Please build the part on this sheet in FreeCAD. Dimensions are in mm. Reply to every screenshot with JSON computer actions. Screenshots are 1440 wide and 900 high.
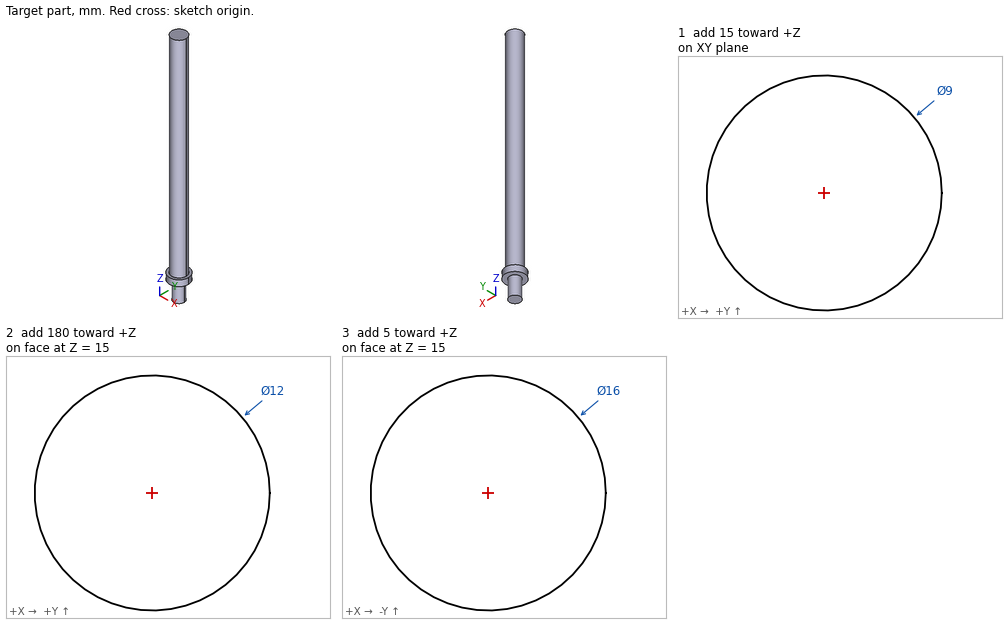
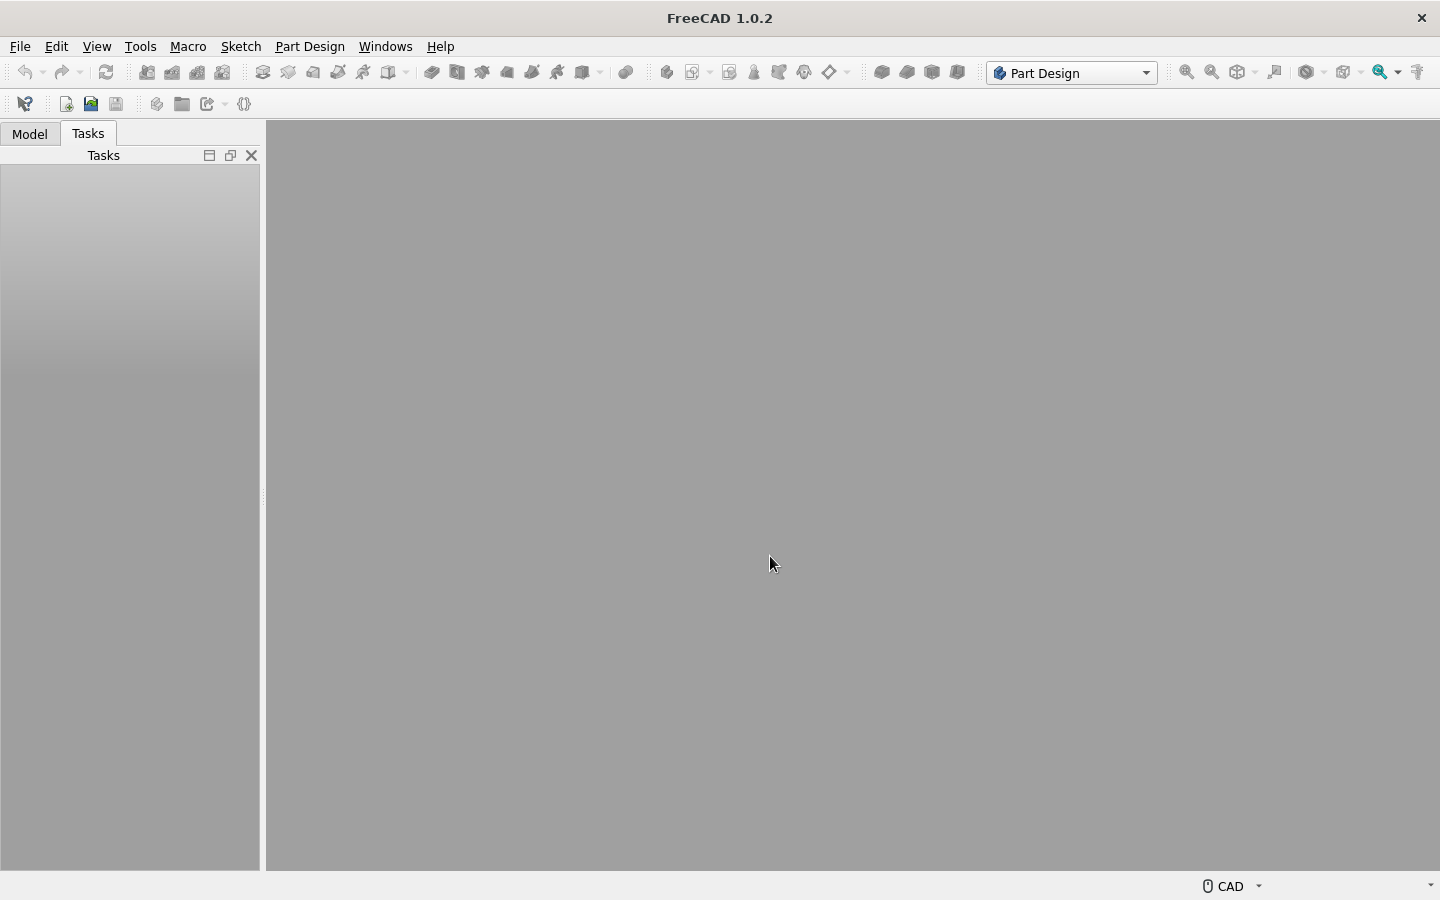
{"action": "key", "text": "ctrl+n"}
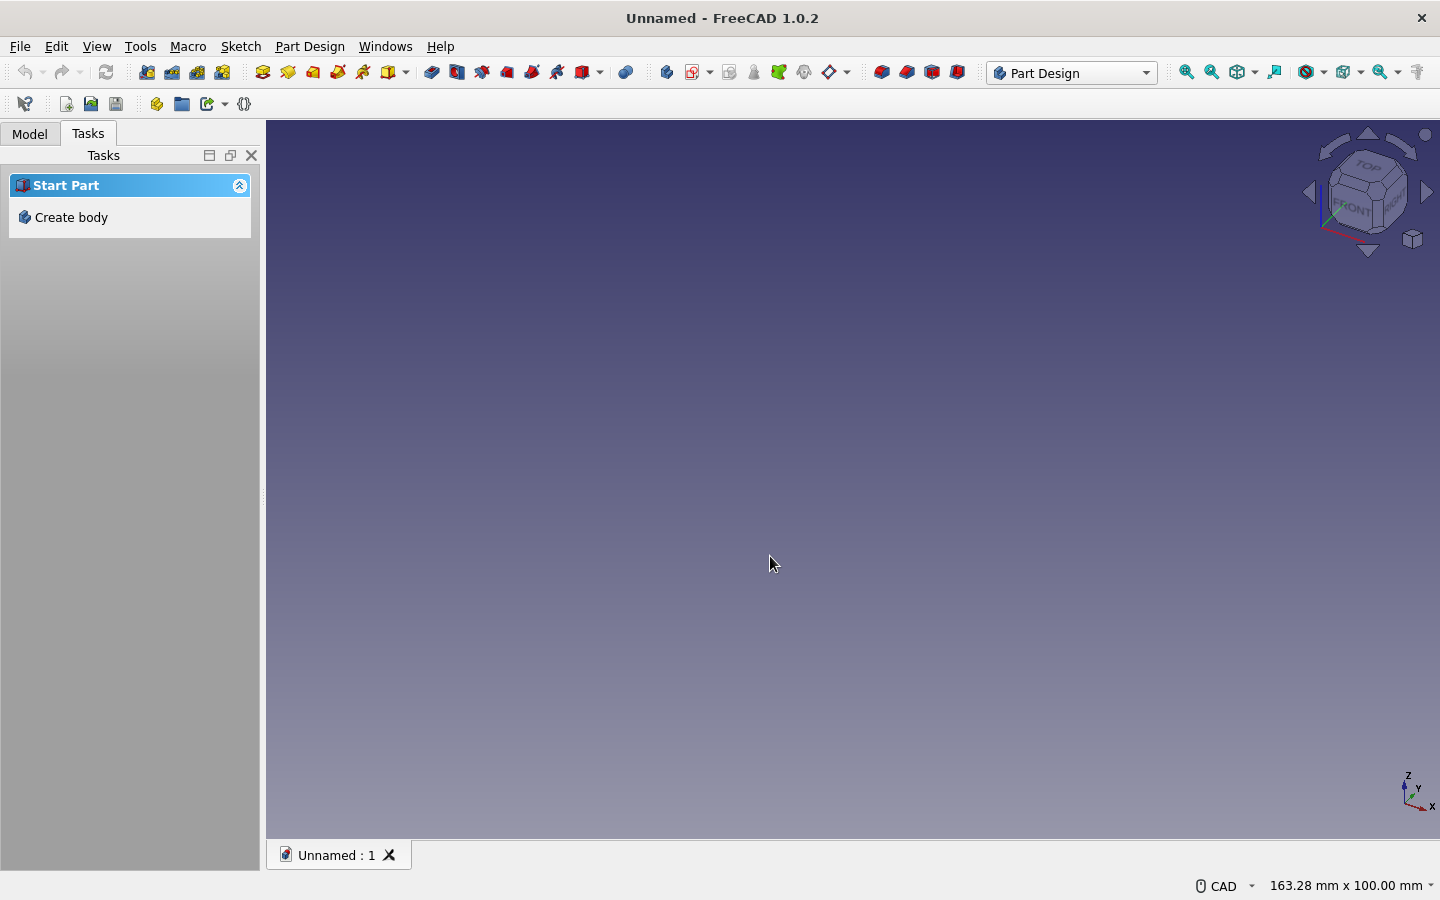
{"action": "left_click", "coordinate": [692, 72]}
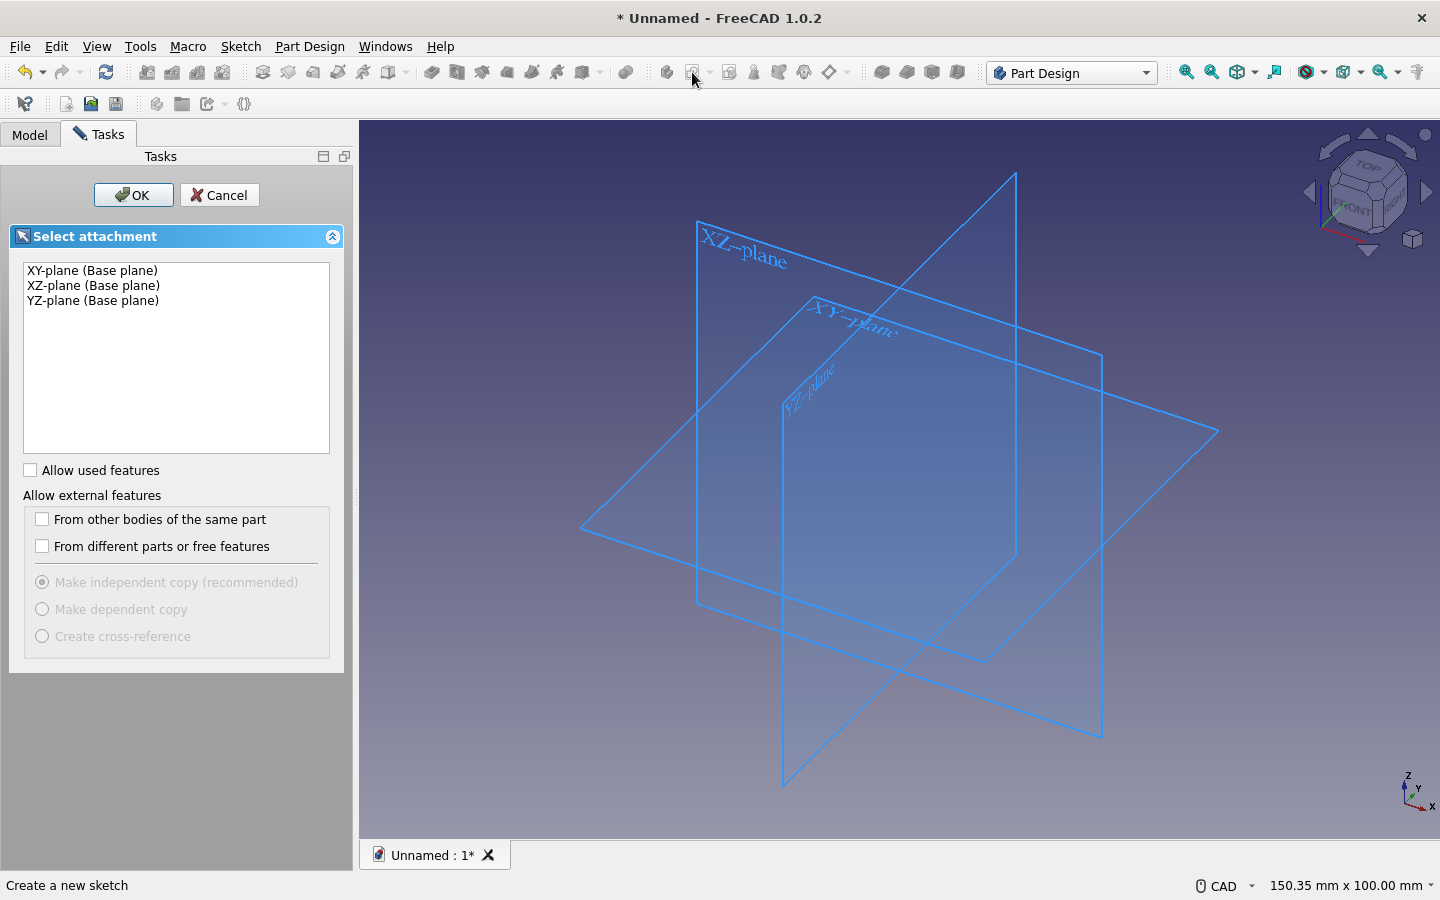
{"action": "left_click", "coordinate": [84, 270]}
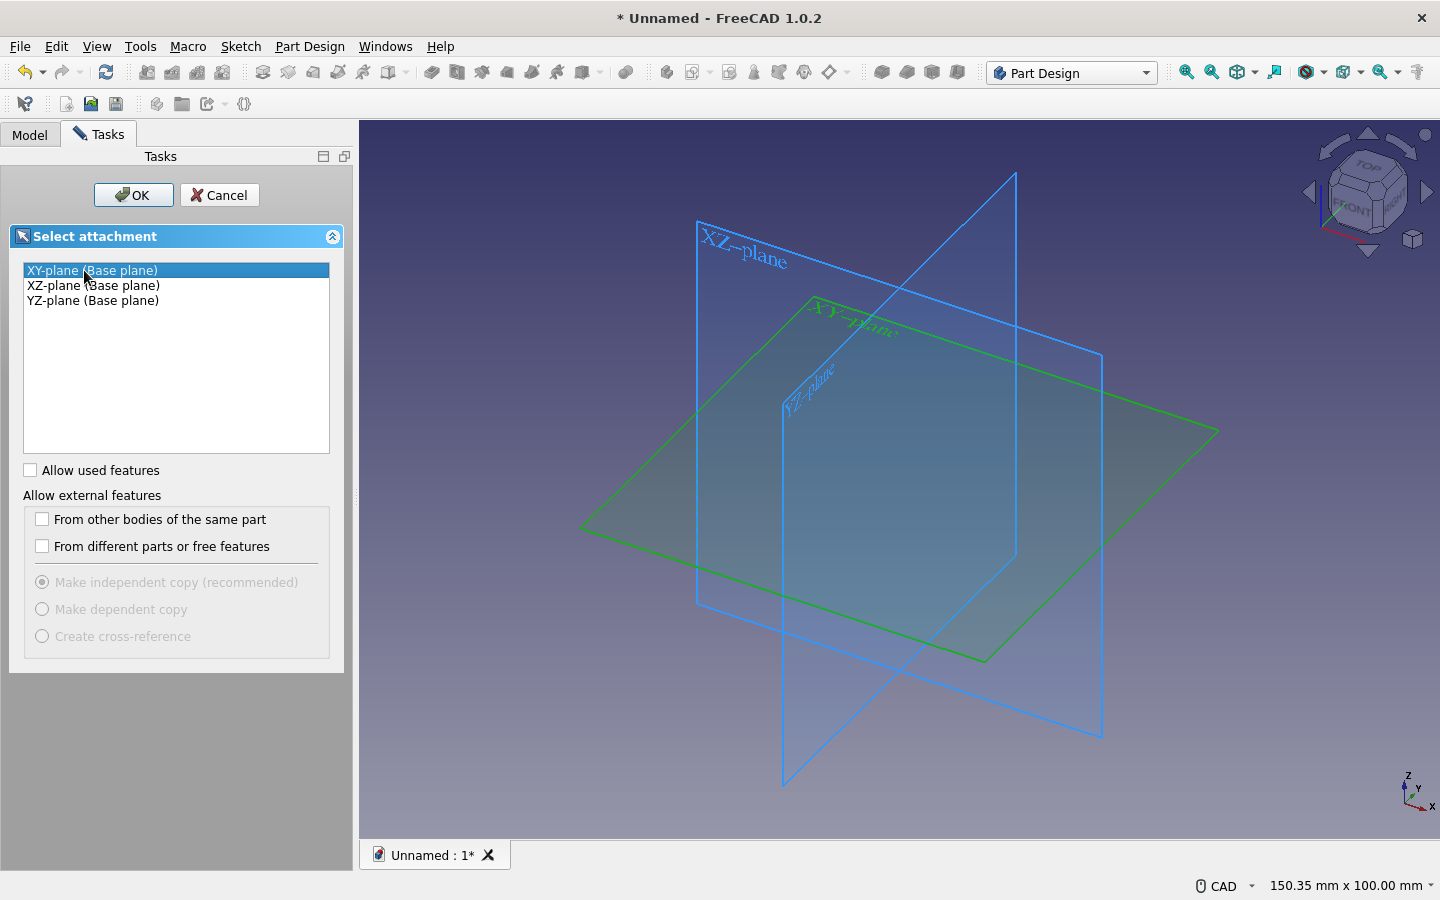
{"action": "left_click", "coordinate": [134, 195]}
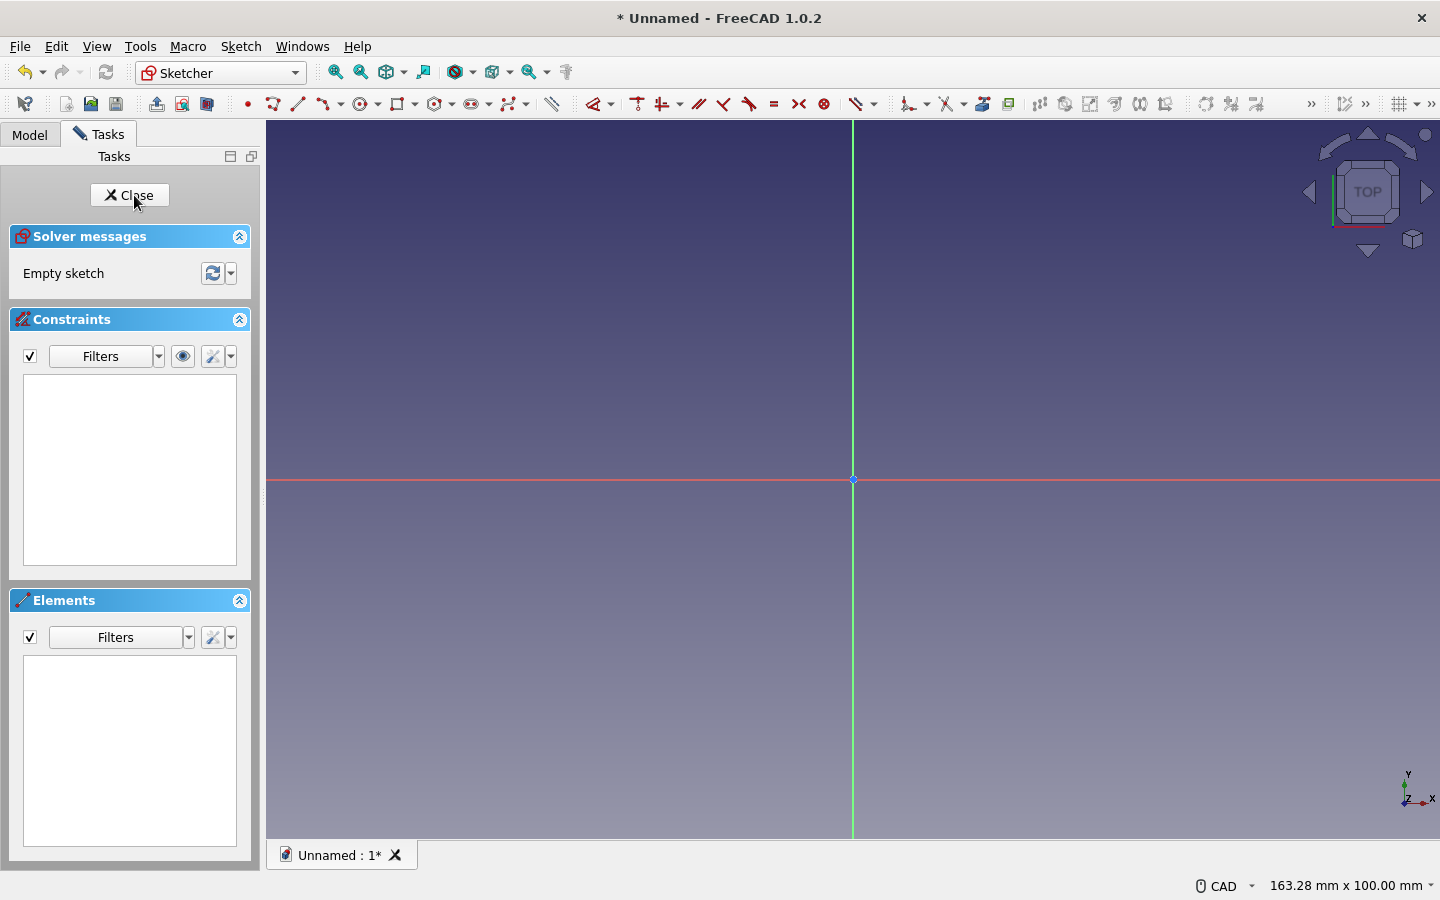
{"action": "scroll", "coordinate": [864, 480], "scroll_direction": "up", "scroll_amount": 10}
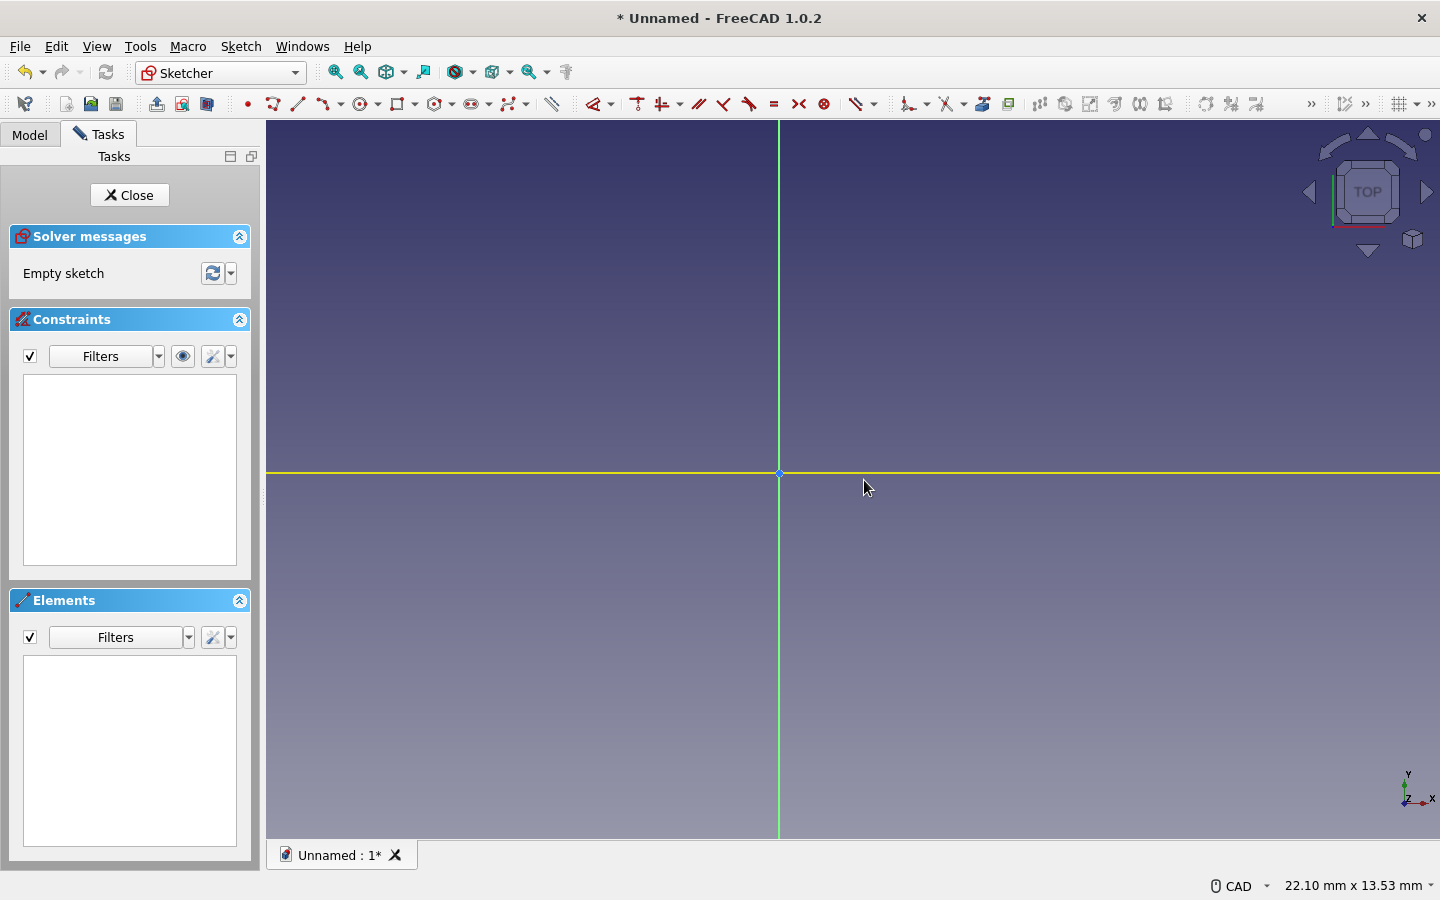
{"action": "left_click", "coordinate": [360, 104]}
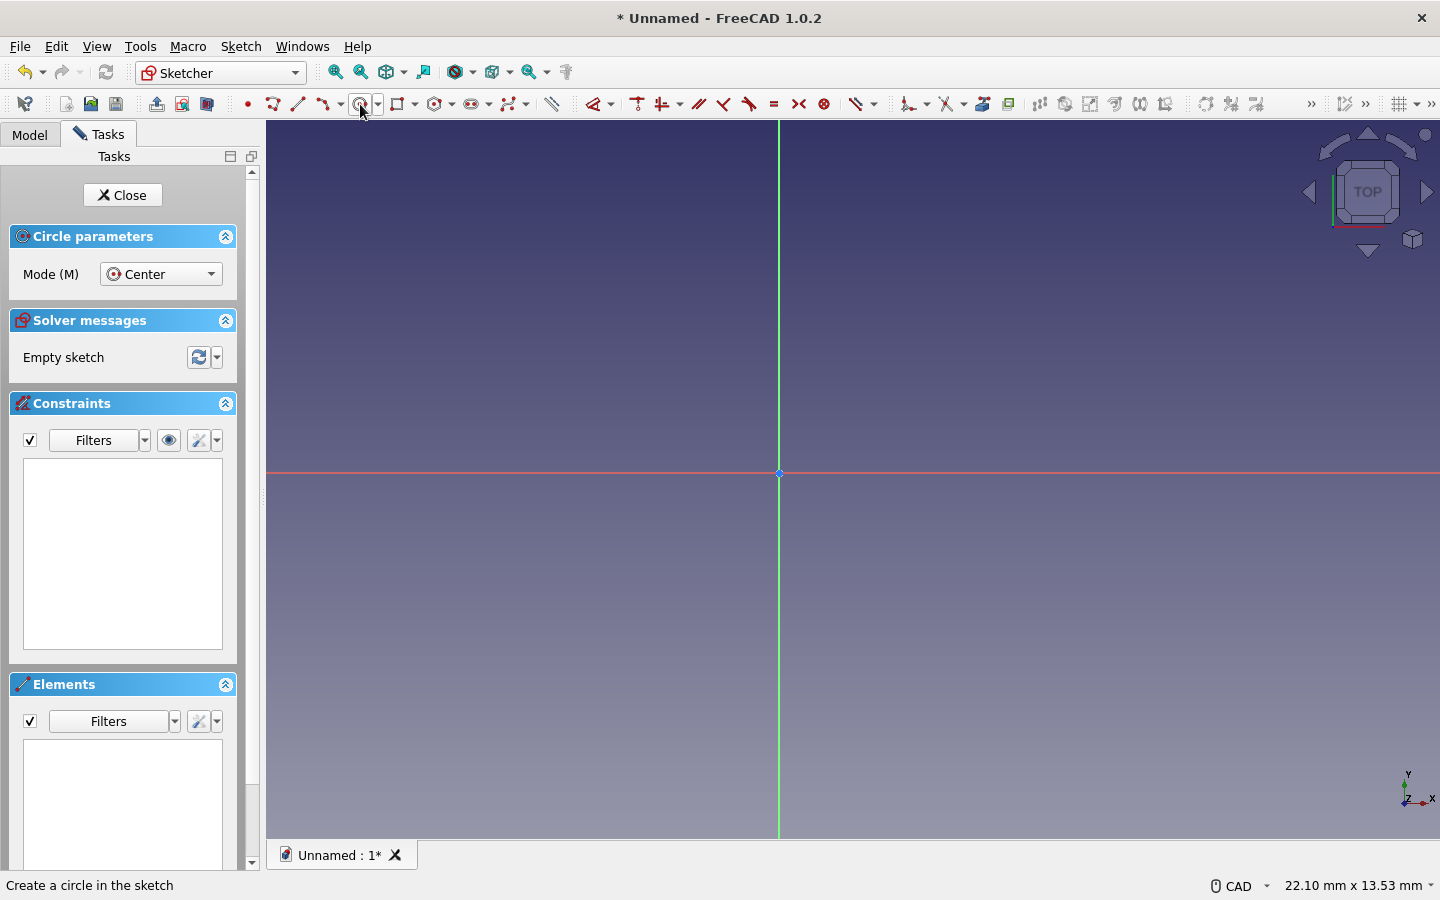
{"action": "left_click", "coordinate": [779, 473]}
{"action": "left_click", "coordinate": [949, 304]}
{"action": "key", "text": "Escape"}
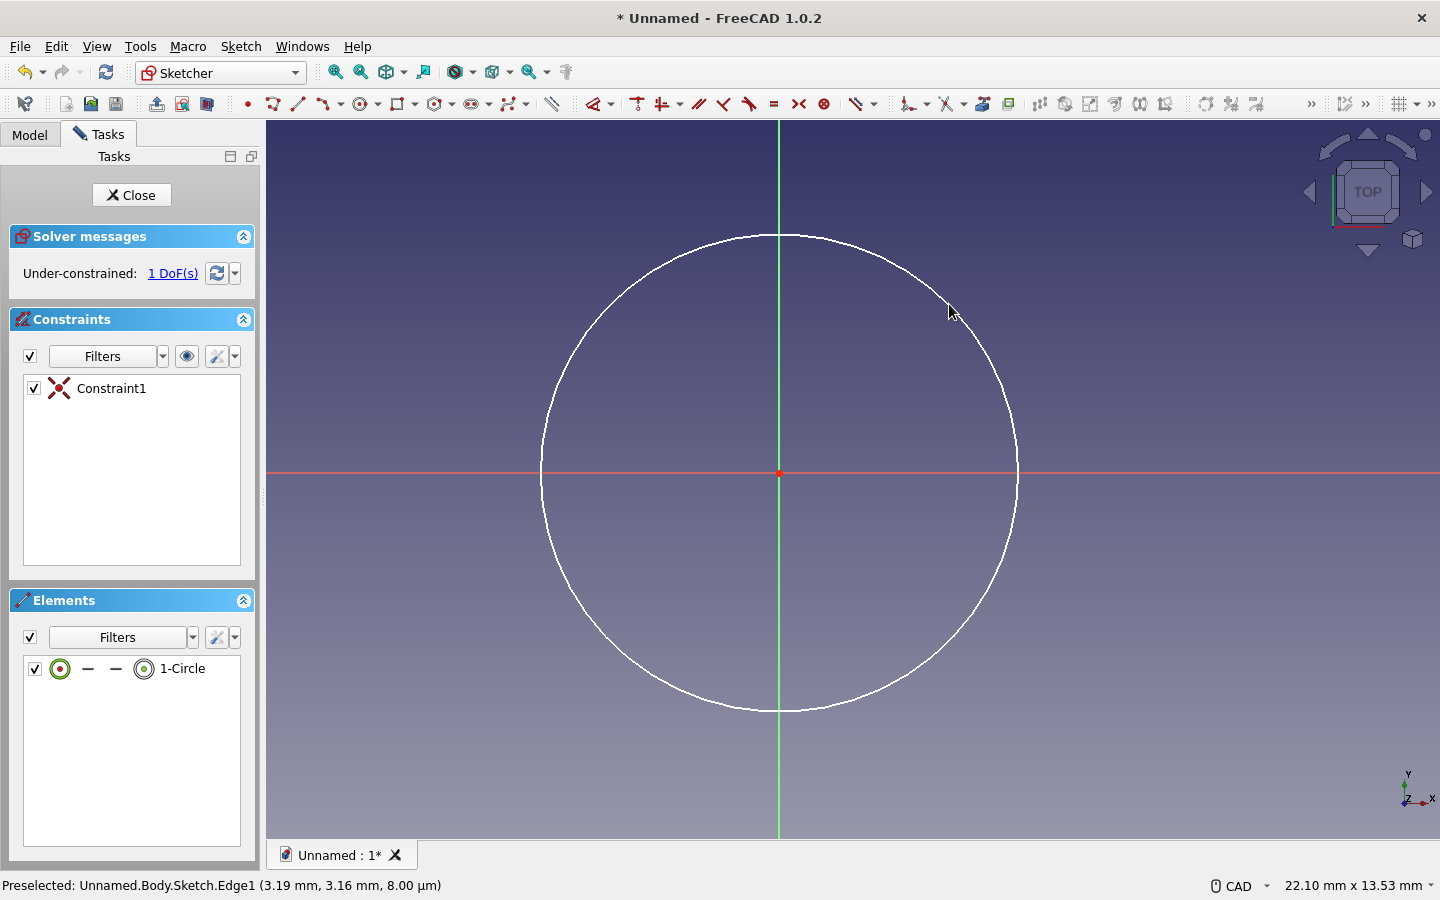
{"action": "left_click", "coordinate": [592, 104]}